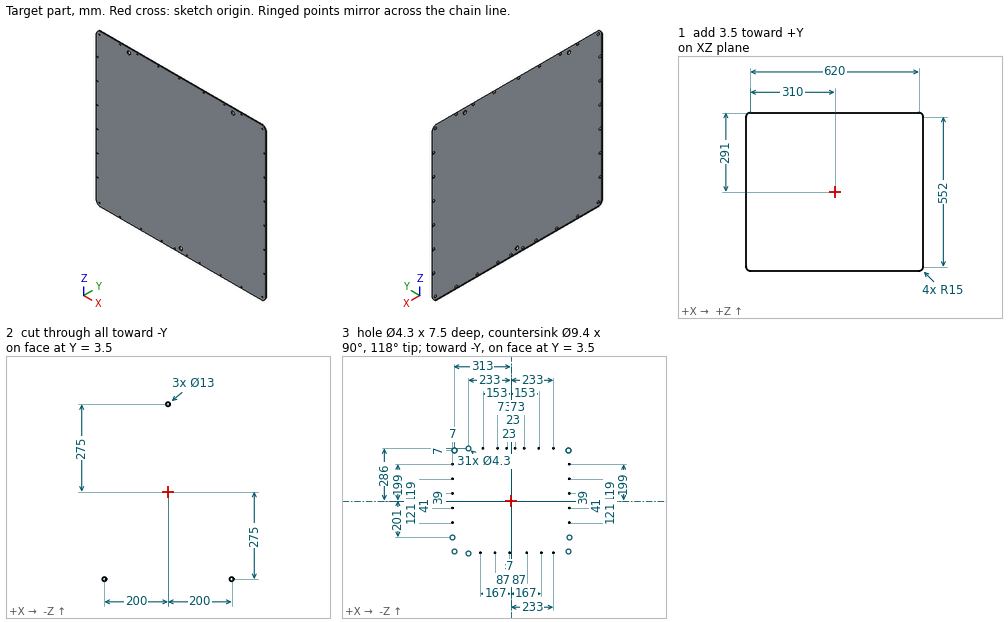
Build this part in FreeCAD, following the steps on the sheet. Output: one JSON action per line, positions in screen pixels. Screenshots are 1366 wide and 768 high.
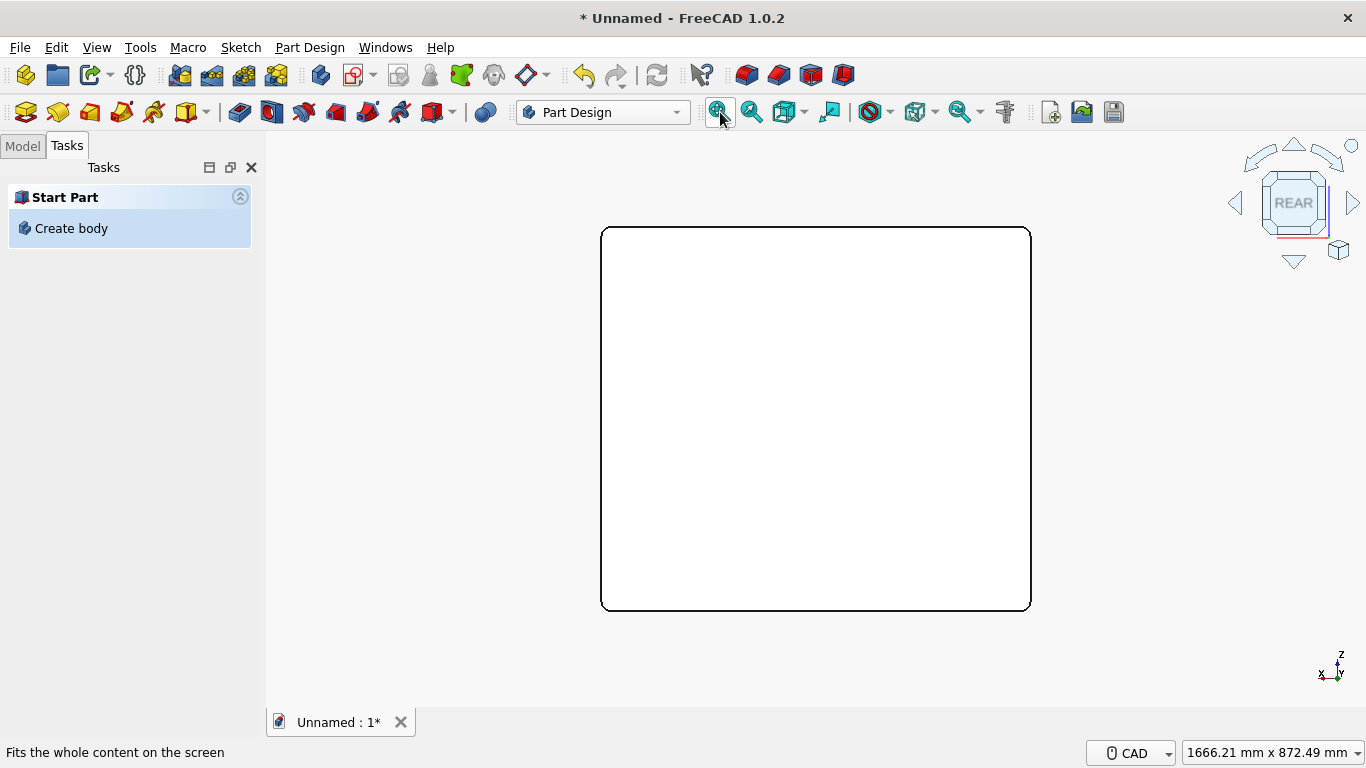
{"action": "left_click", "coordinate": [816, 418]}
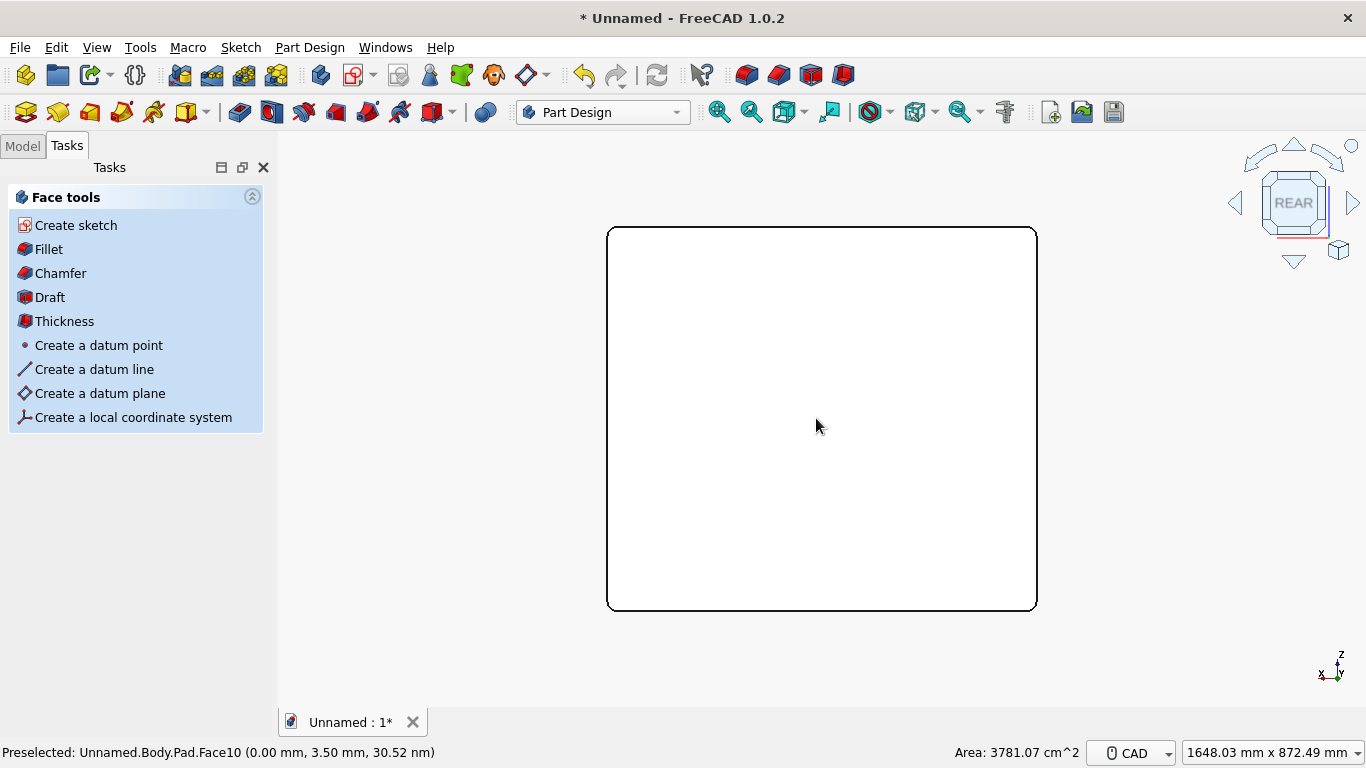
{"action": "left_click", "coordinate": [354, 76]}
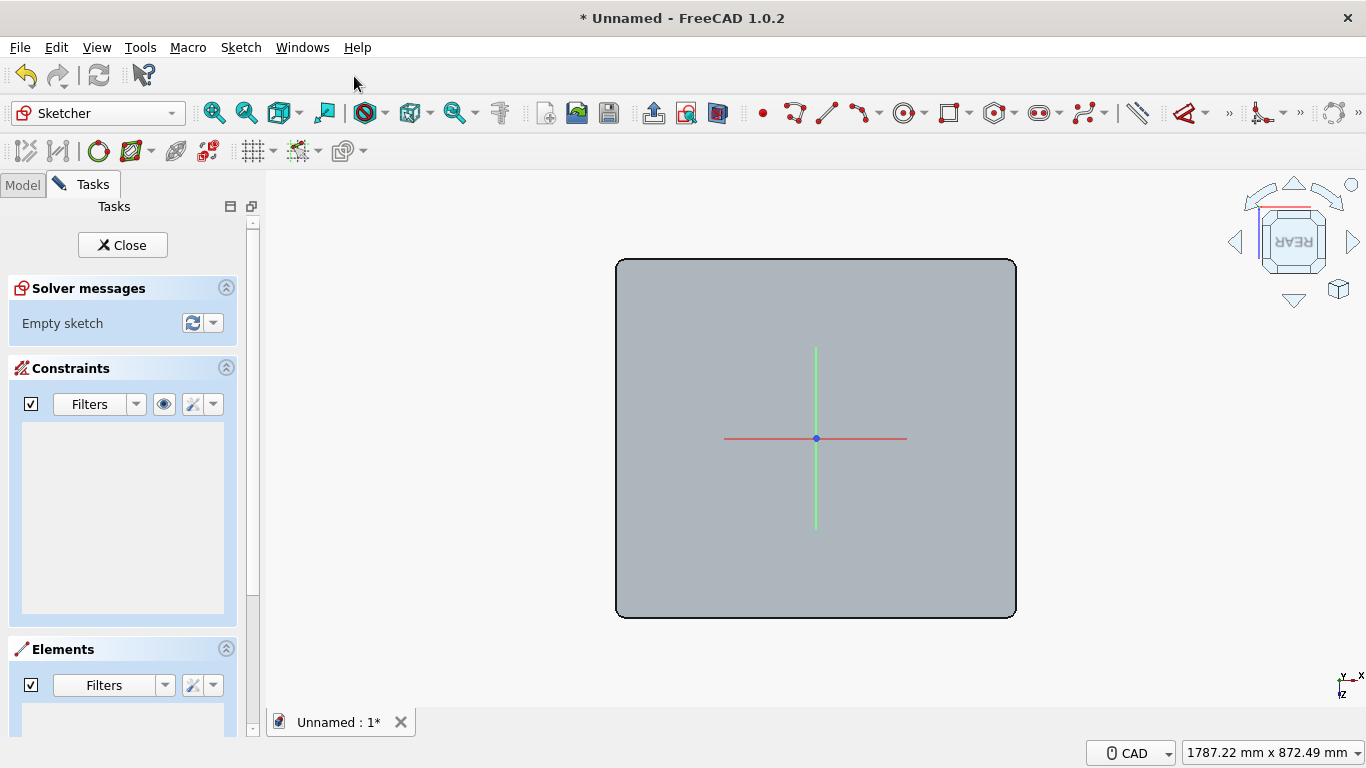
{"action": "left_click", "coordinate": [904, 114]}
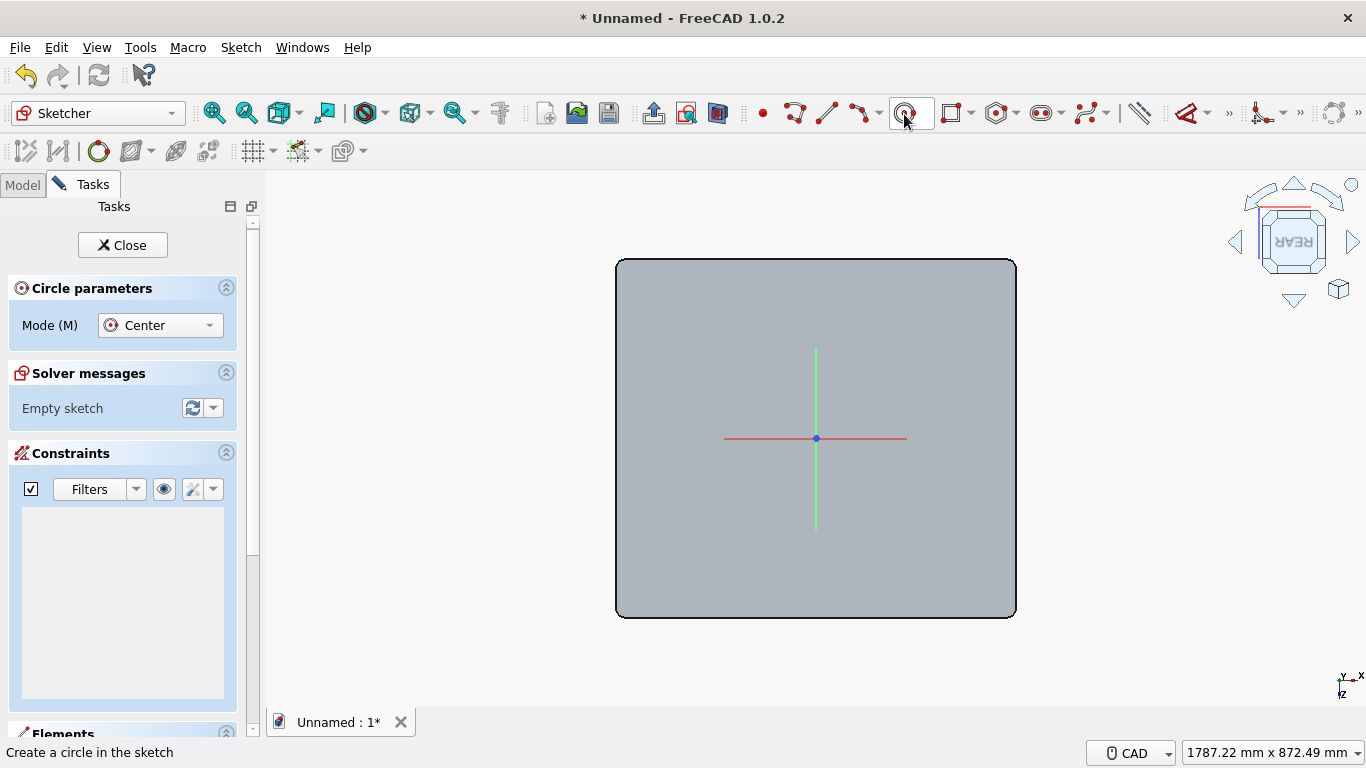
{"action": "scroll", "coordinate": [816, 269], "scroll_direction": "up", "scroll_amount": 9}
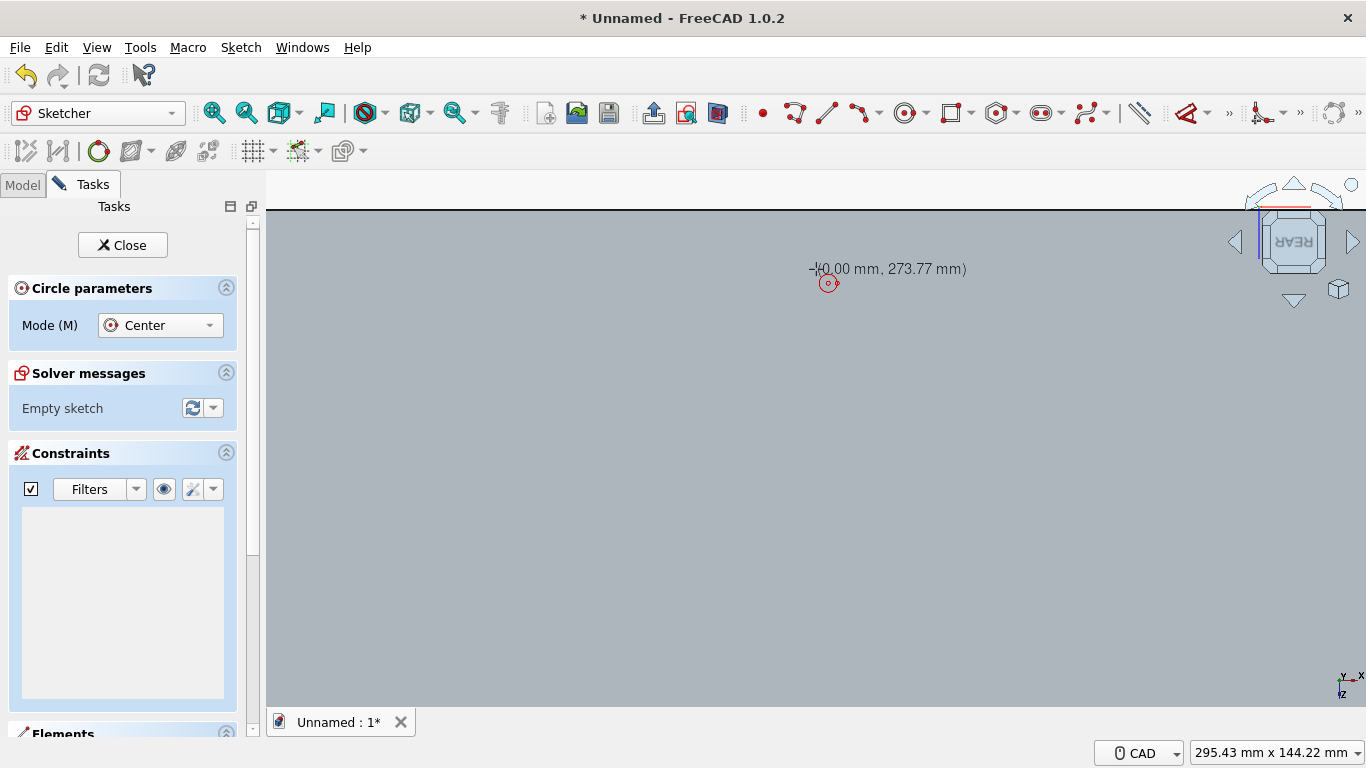
{"action": "scroll", "coordinate": [734, 269], "scroll_direction": "down", "scroll_amount": 9}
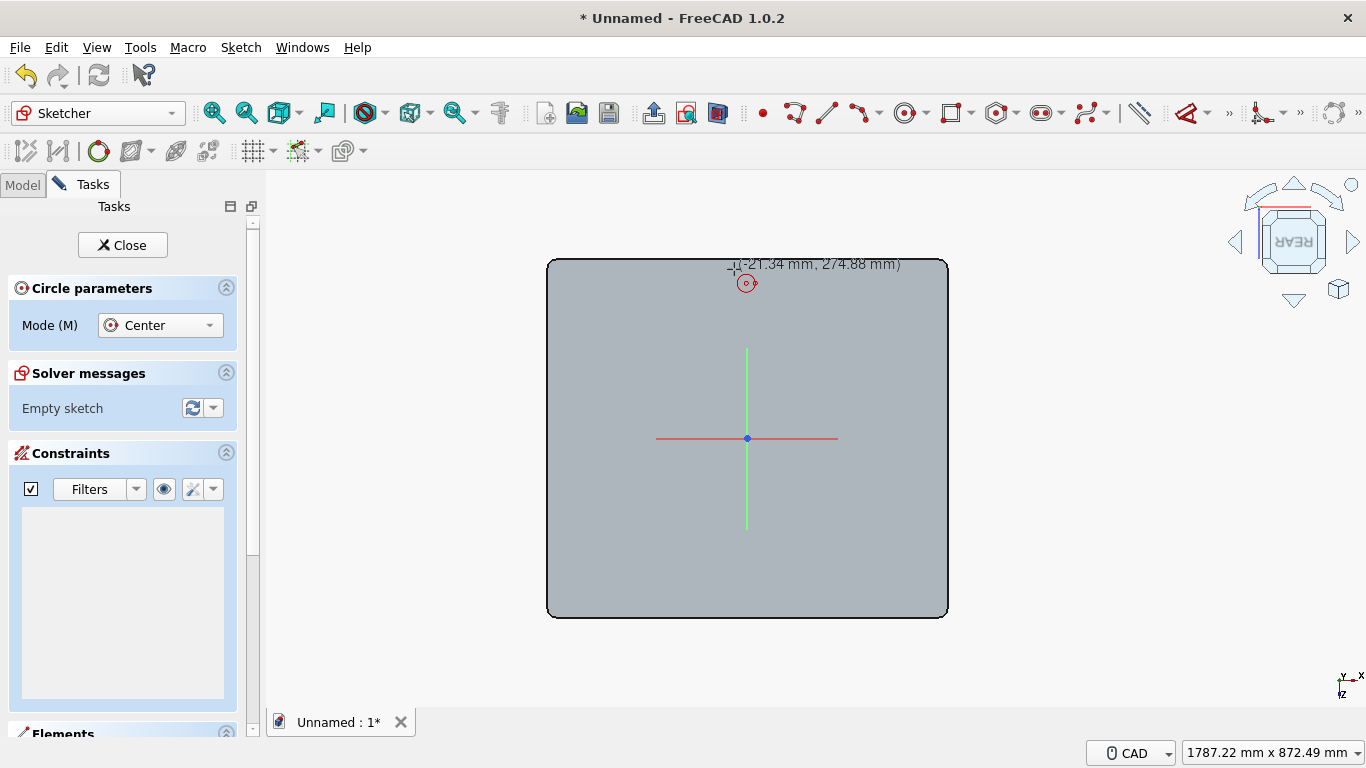
{"action": "left_click", "coordinate": [747, 269]}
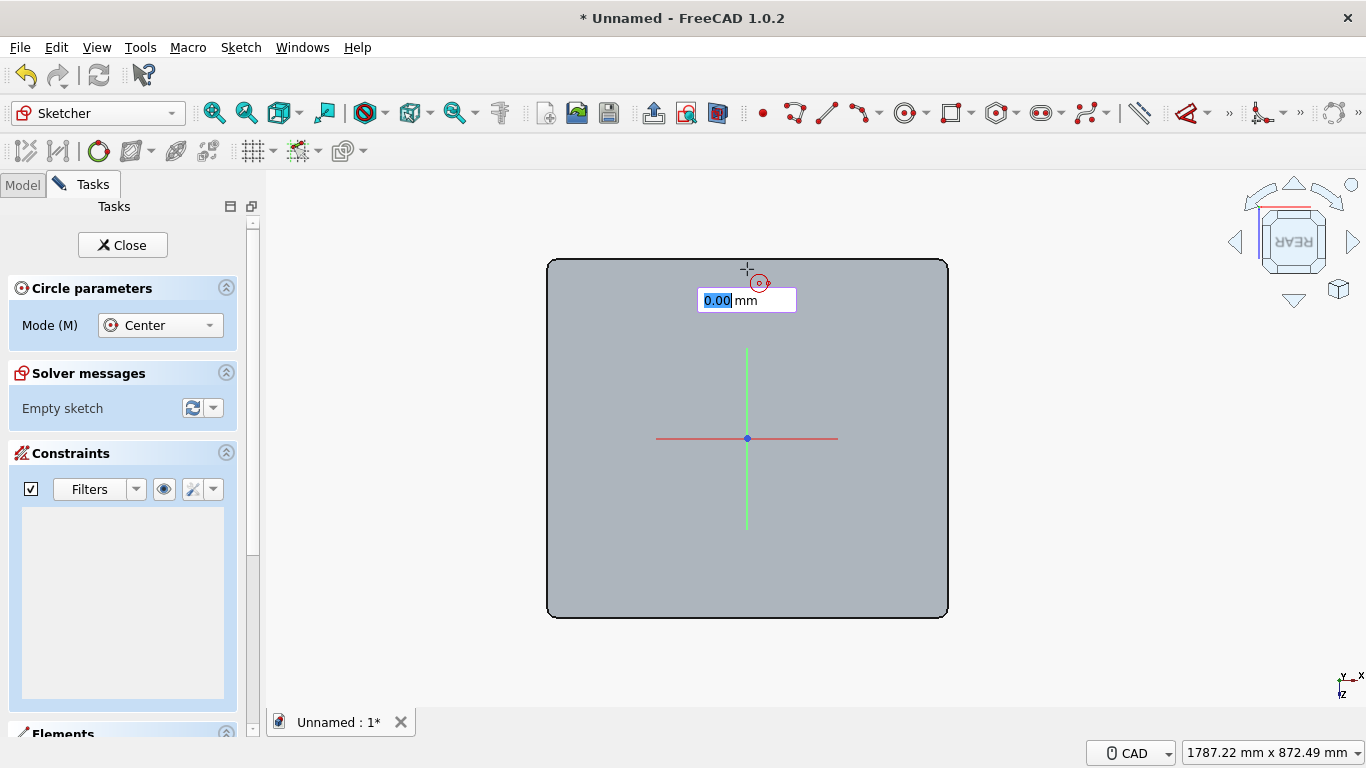
{"action": "scroll", "coordinate": [751, 268], "scroll_direction": "up", "scroll_amount": 8}
{"action": "mouse_move", "coordinate": [751, 267]}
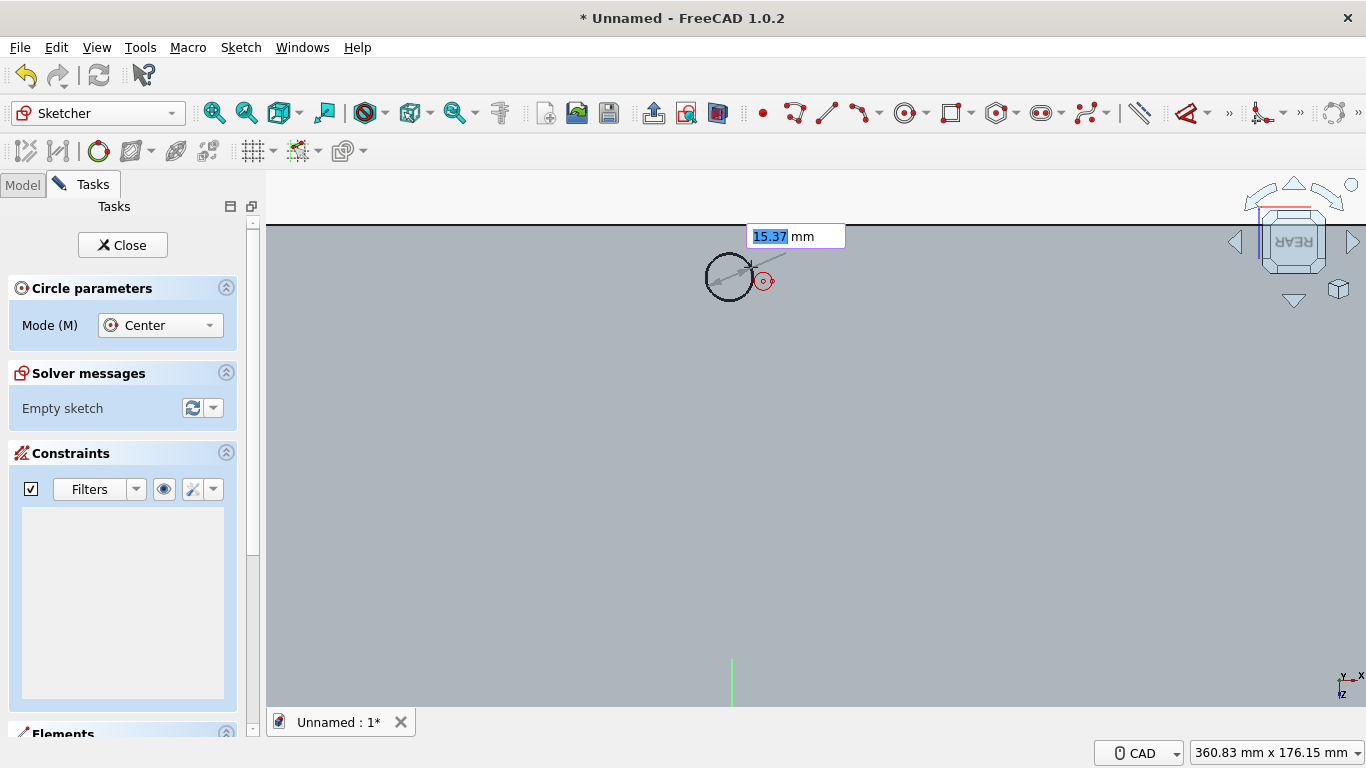
{"action": "type", "text": "13"}
{"action": "key", "text": "Return"}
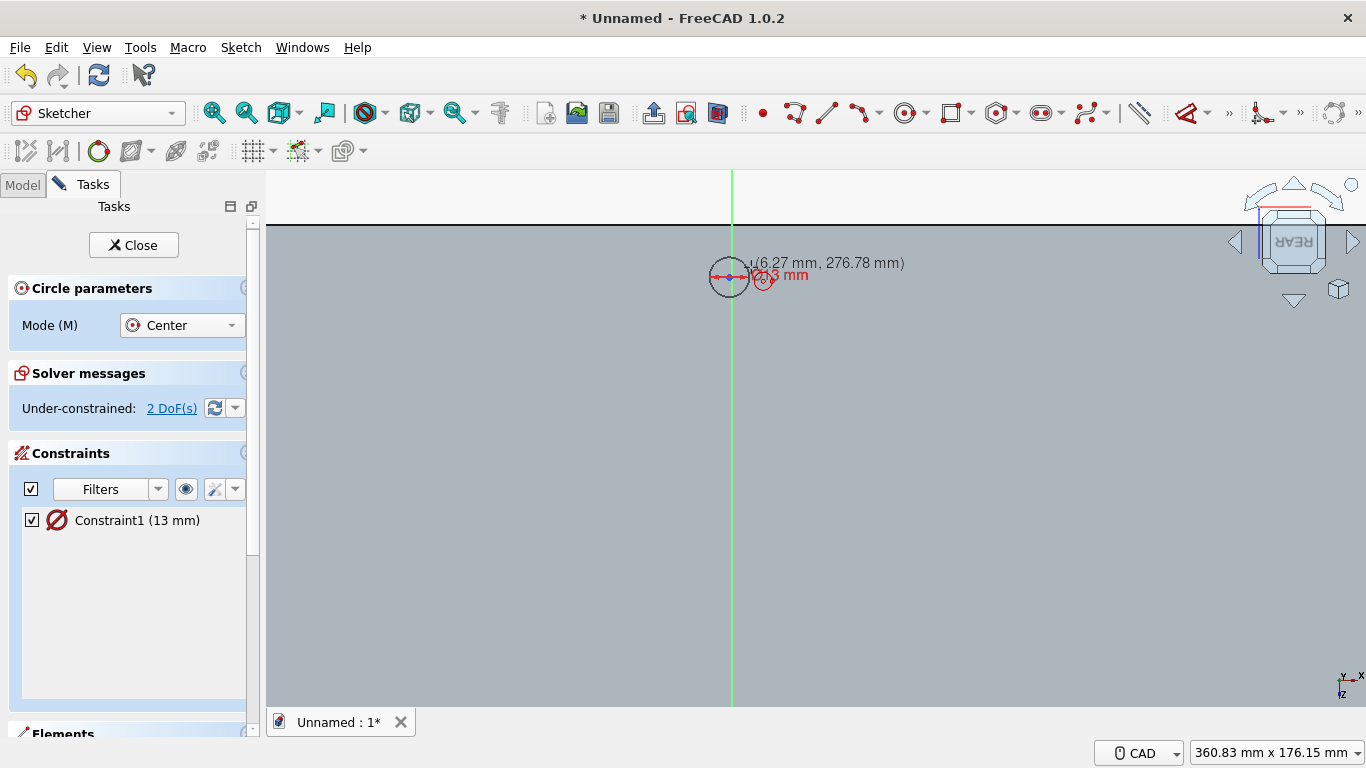
{"action": "scroll", "coordinate": [751, 268], "scroll_direction": "down", "scroll_amount": 8}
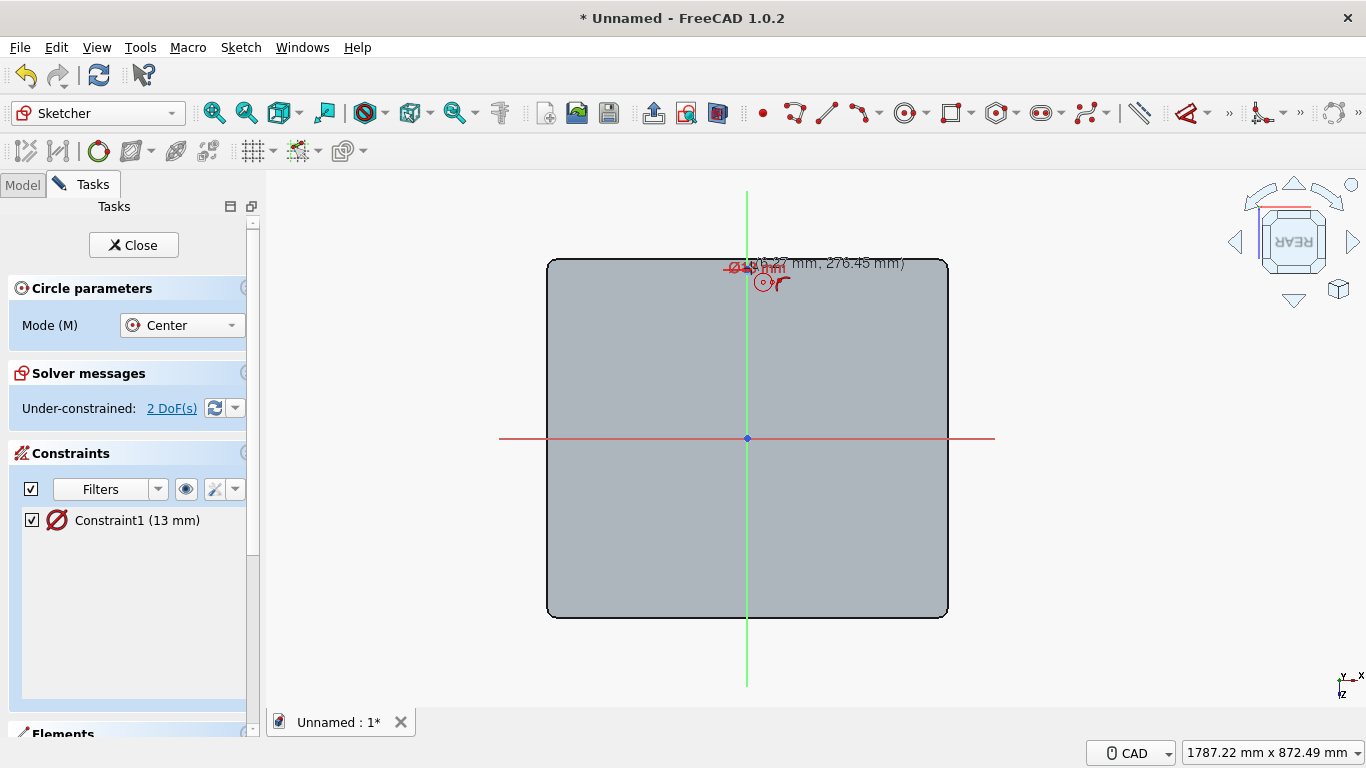
{"action": "scroll", "coordinate": [871, 608], "scroll_direction": "up", "scroll_amount": 9}